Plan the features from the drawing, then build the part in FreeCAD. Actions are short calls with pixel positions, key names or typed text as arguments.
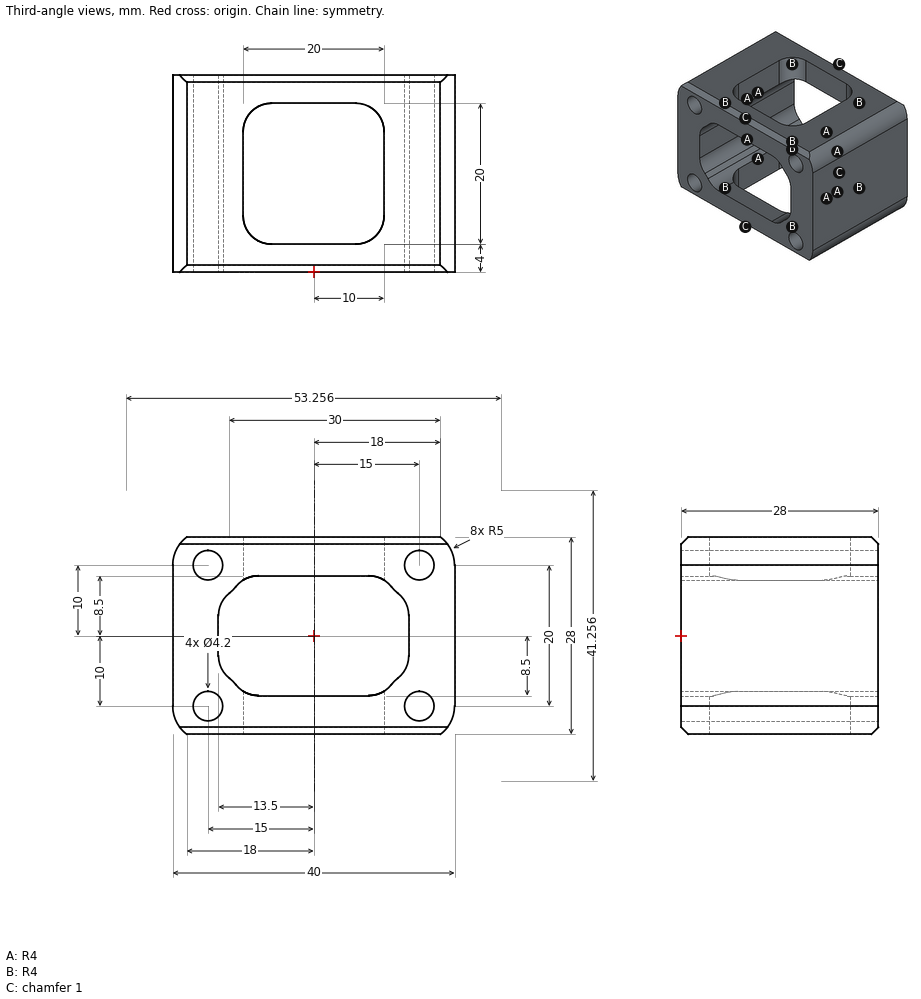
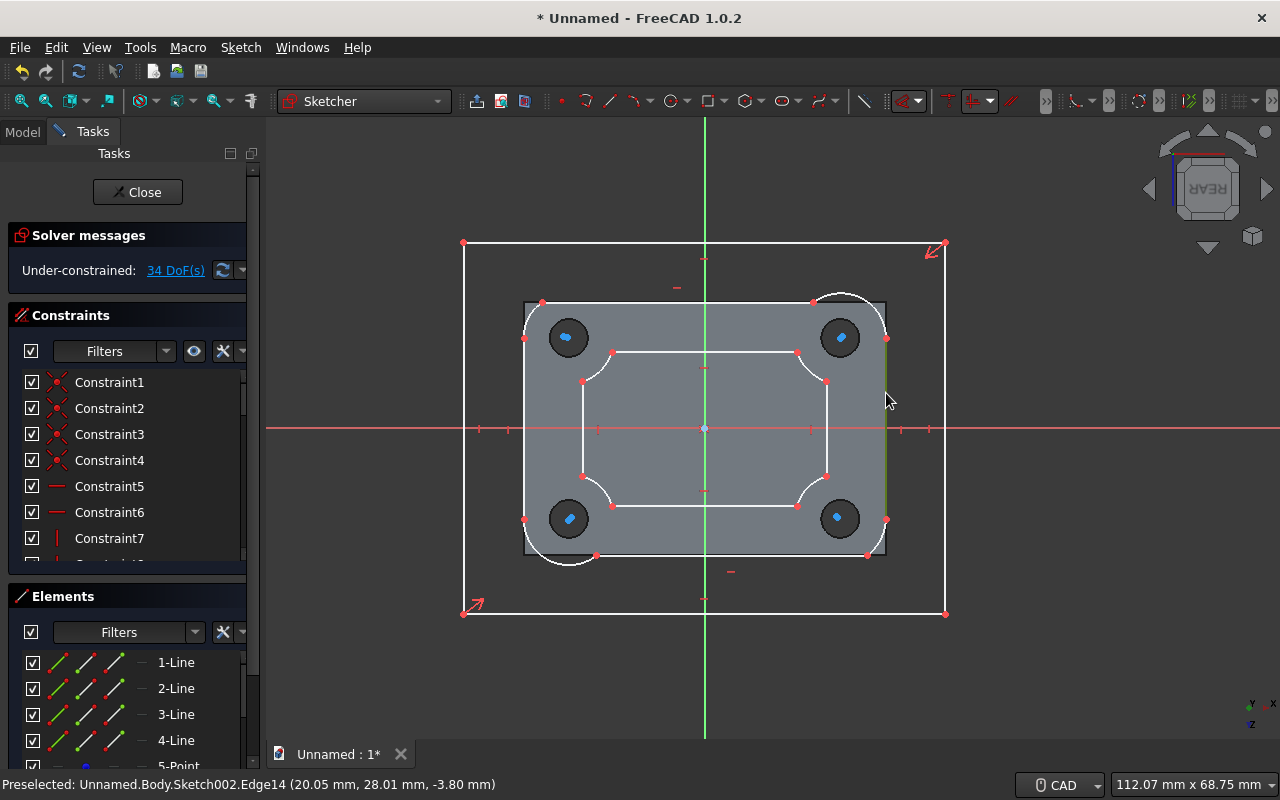
click(876, 547)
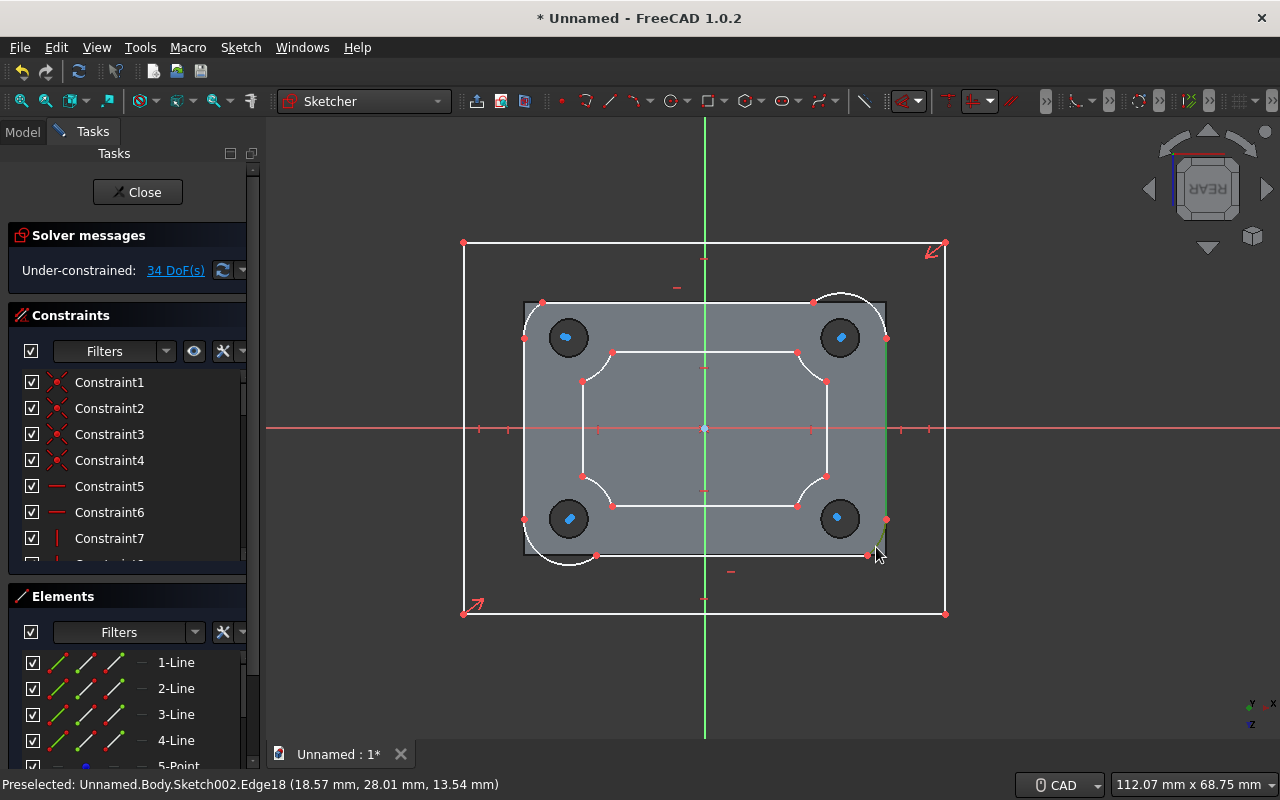
key(t)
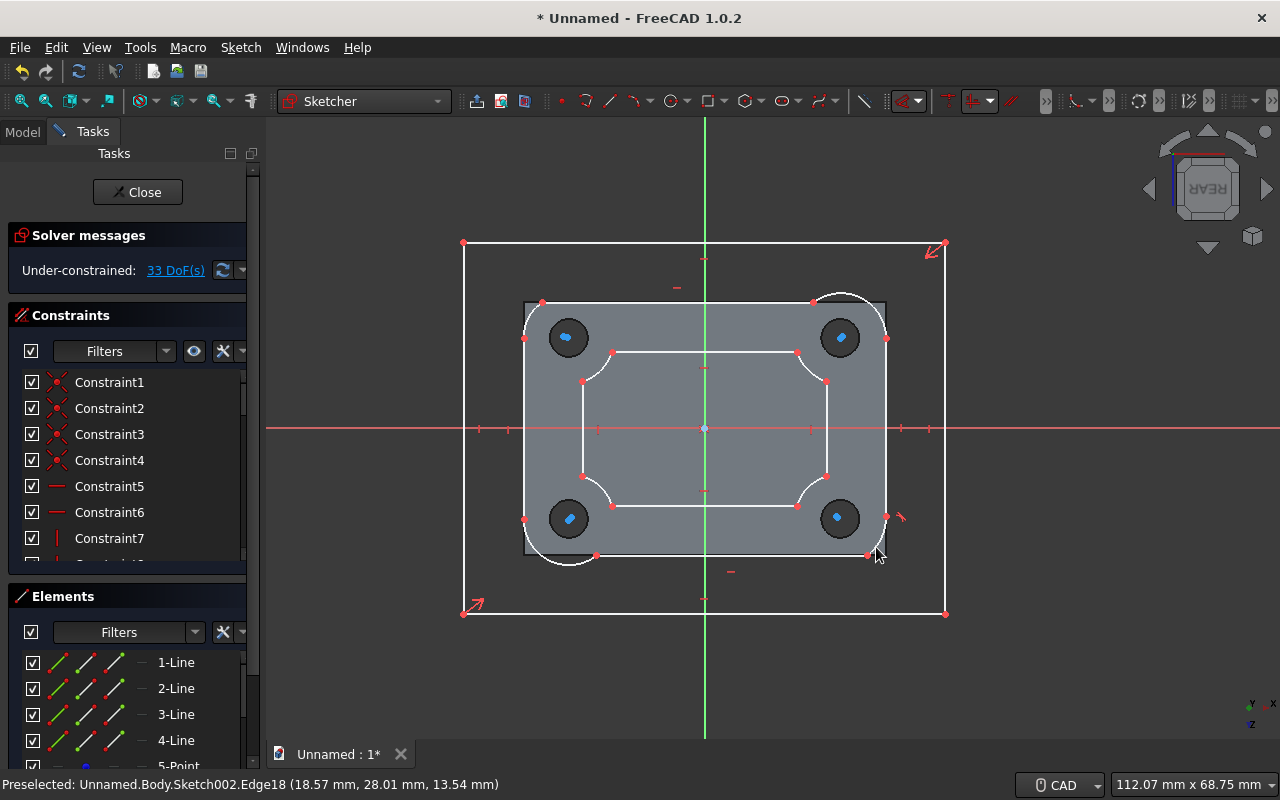
click(886, 392)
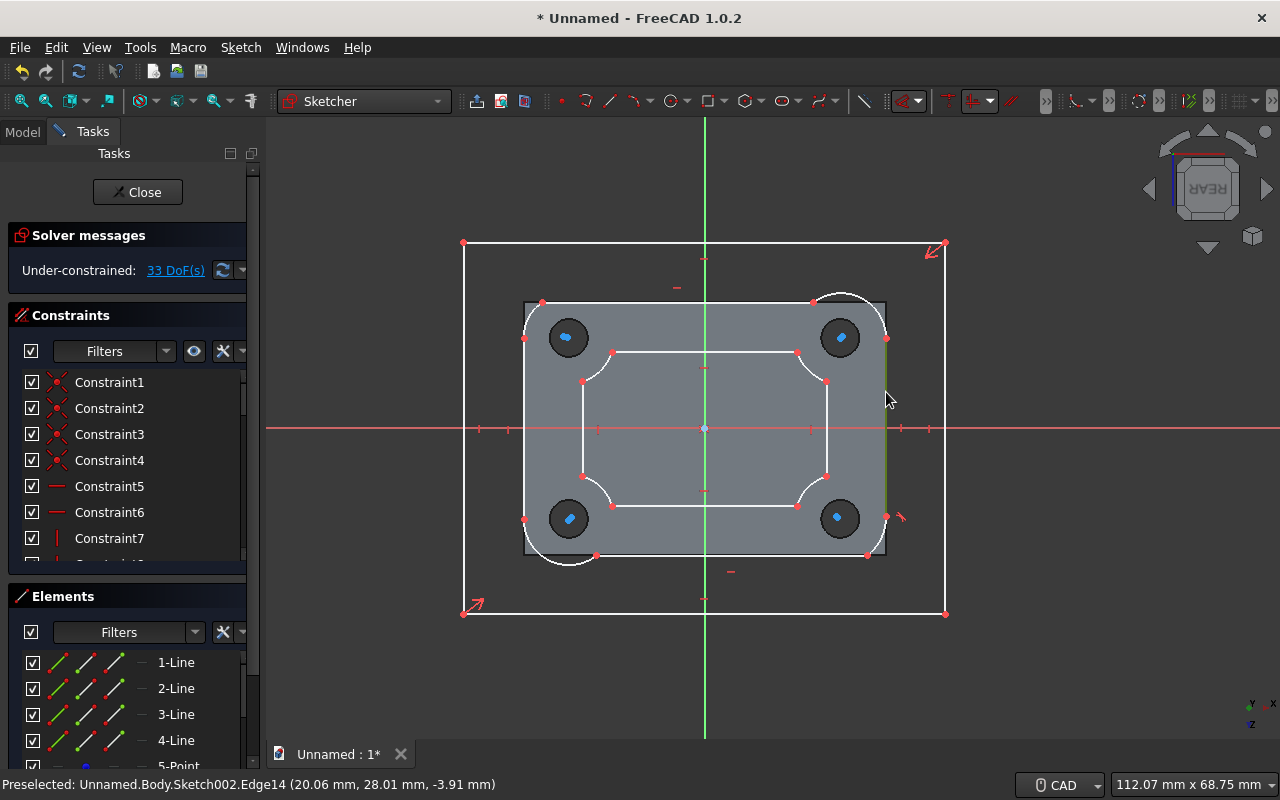
click(877, 311)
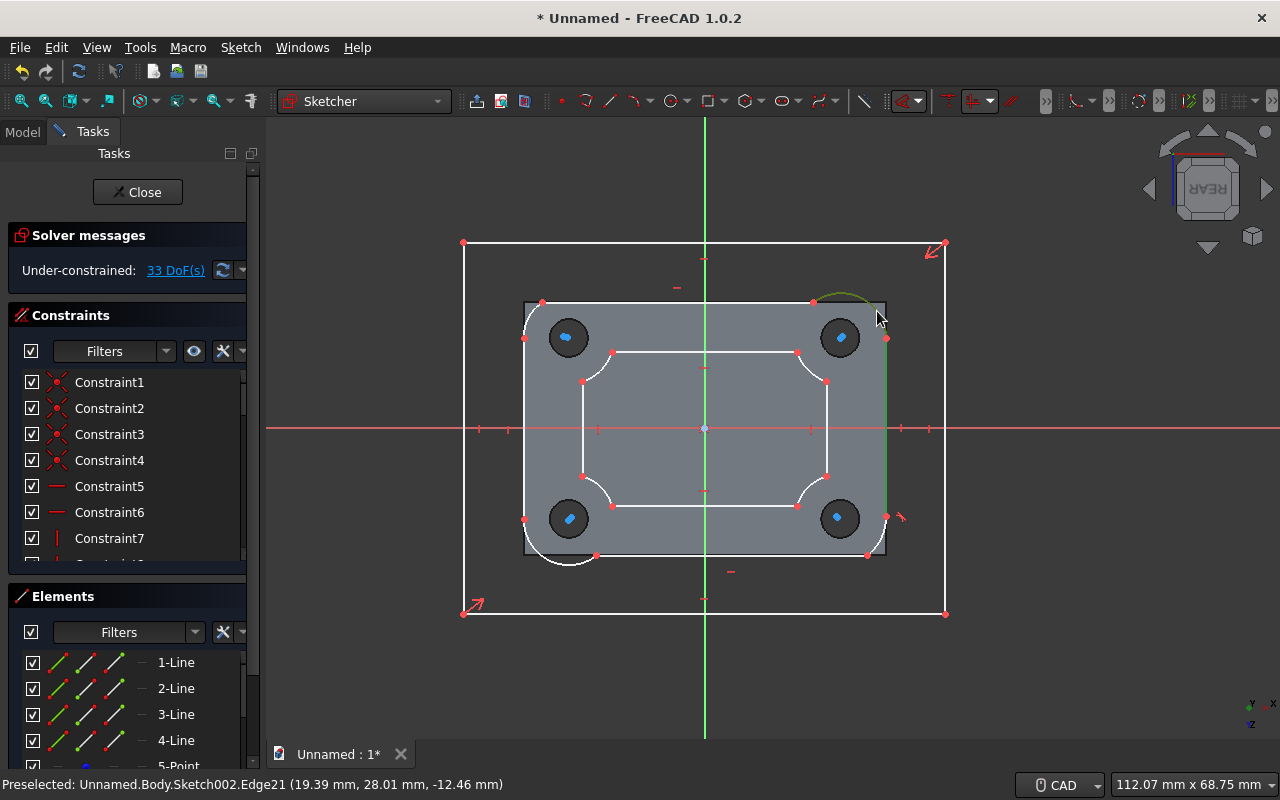
key(t)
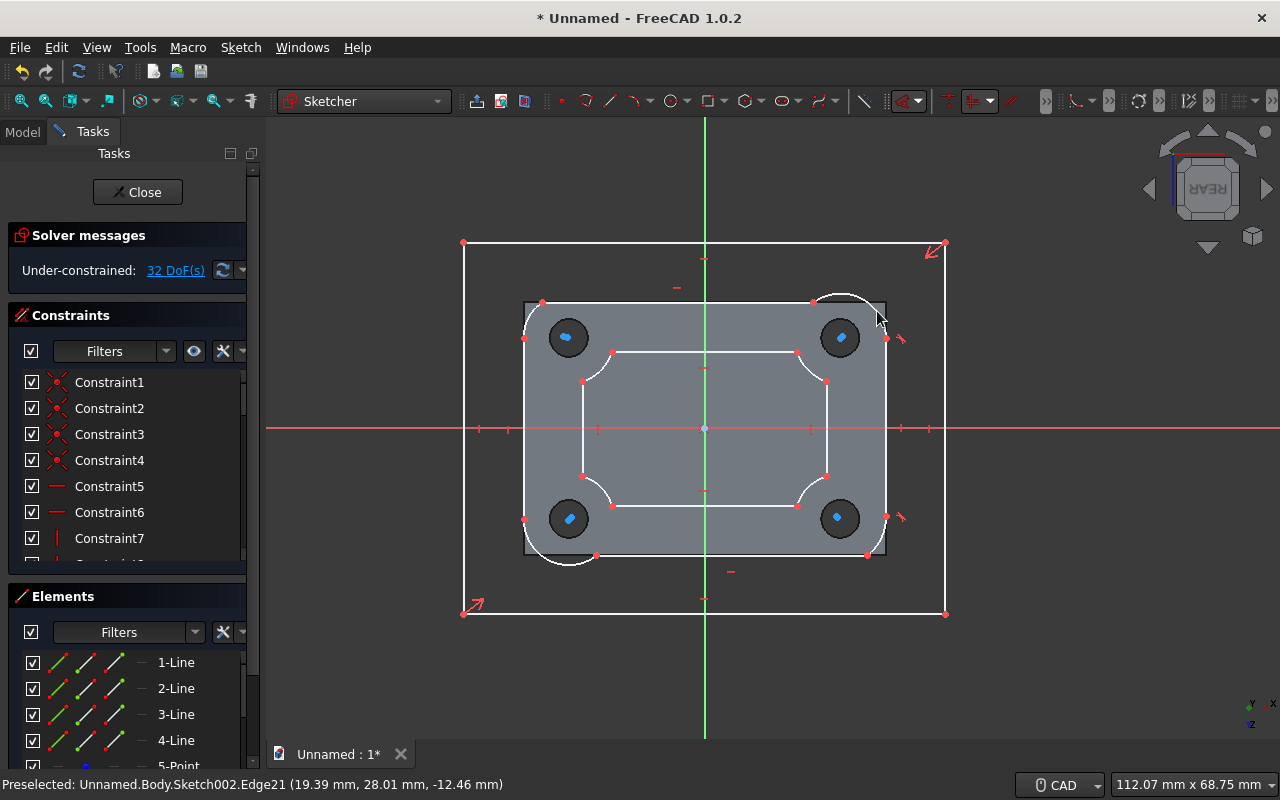
click(524, 466)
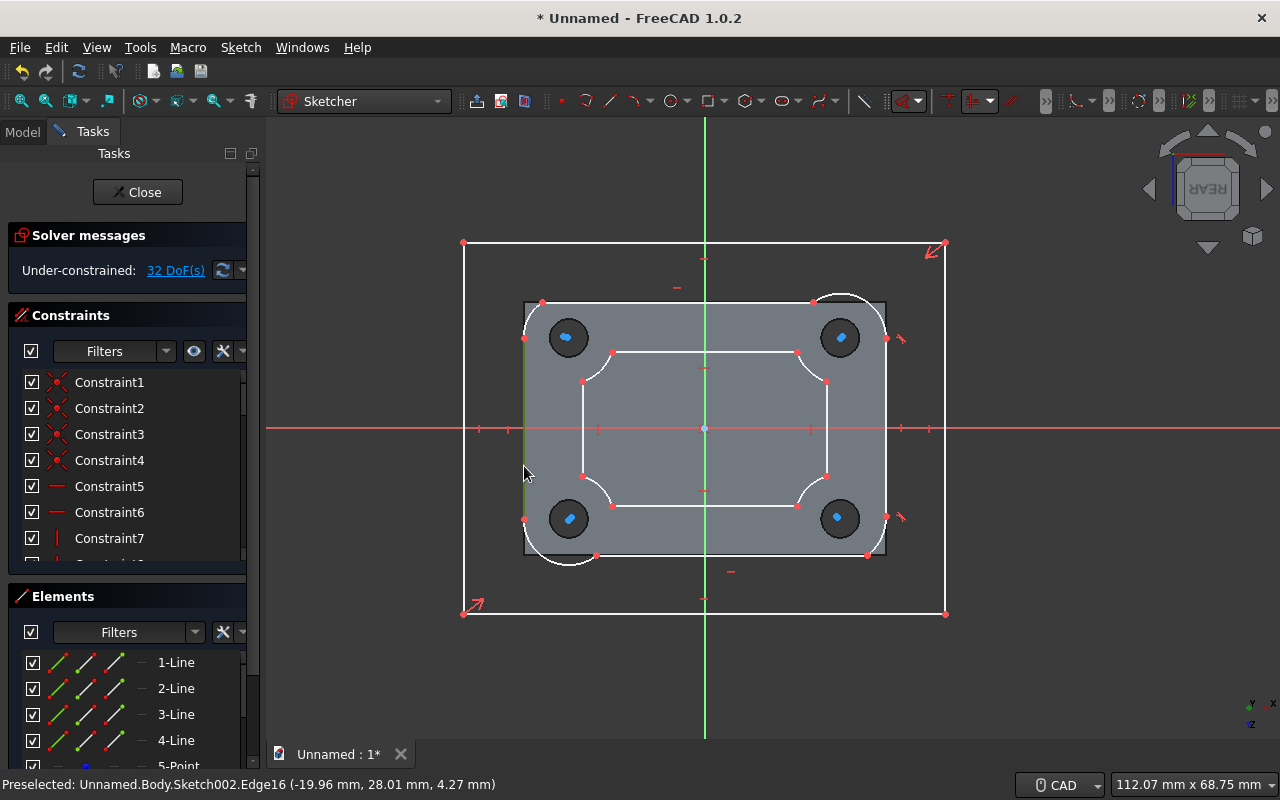
click(534, 548)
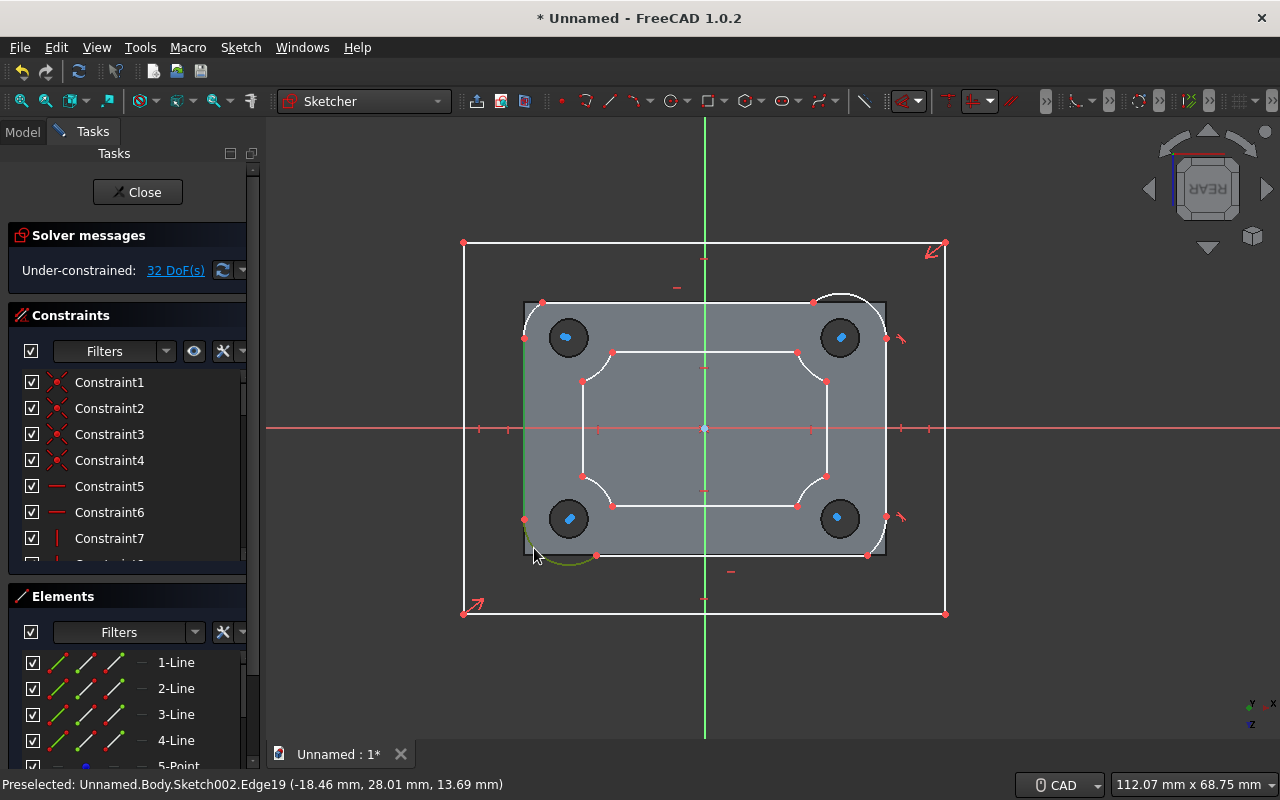
key(t)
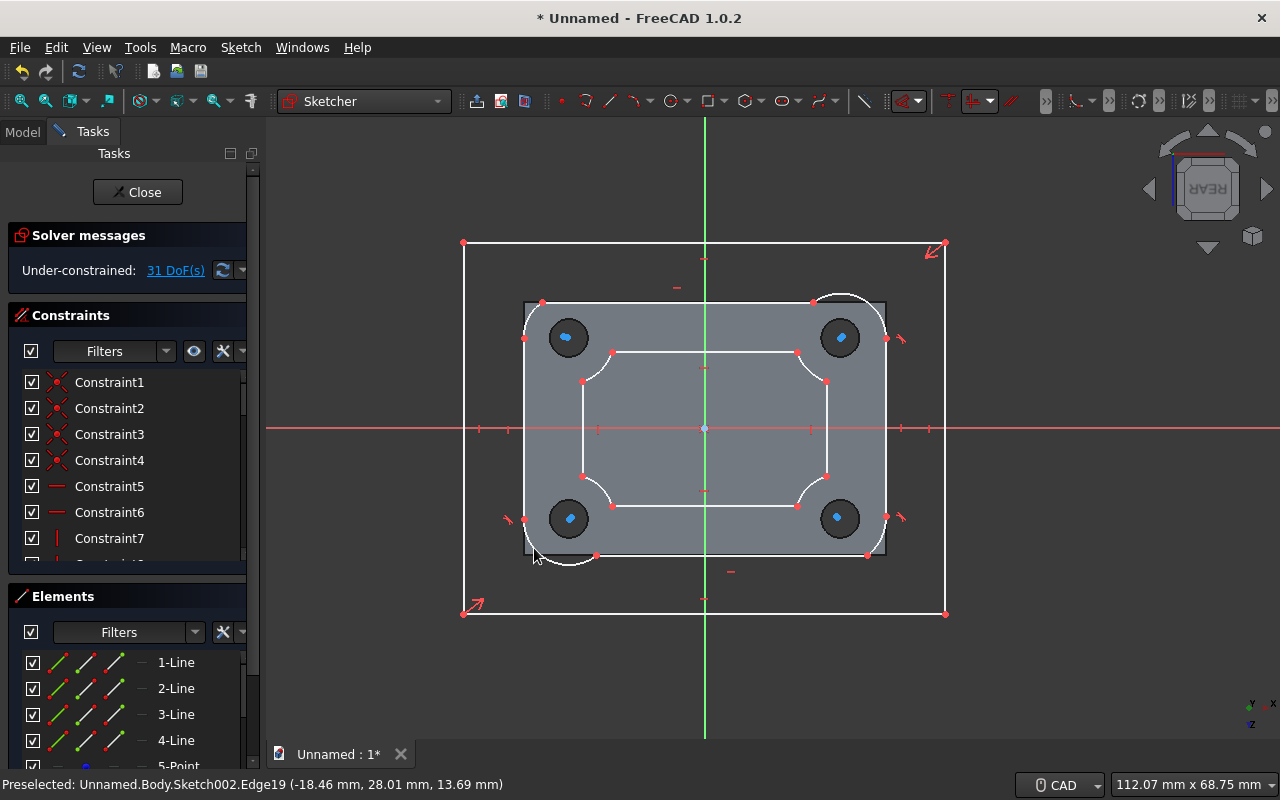
click(524, 466)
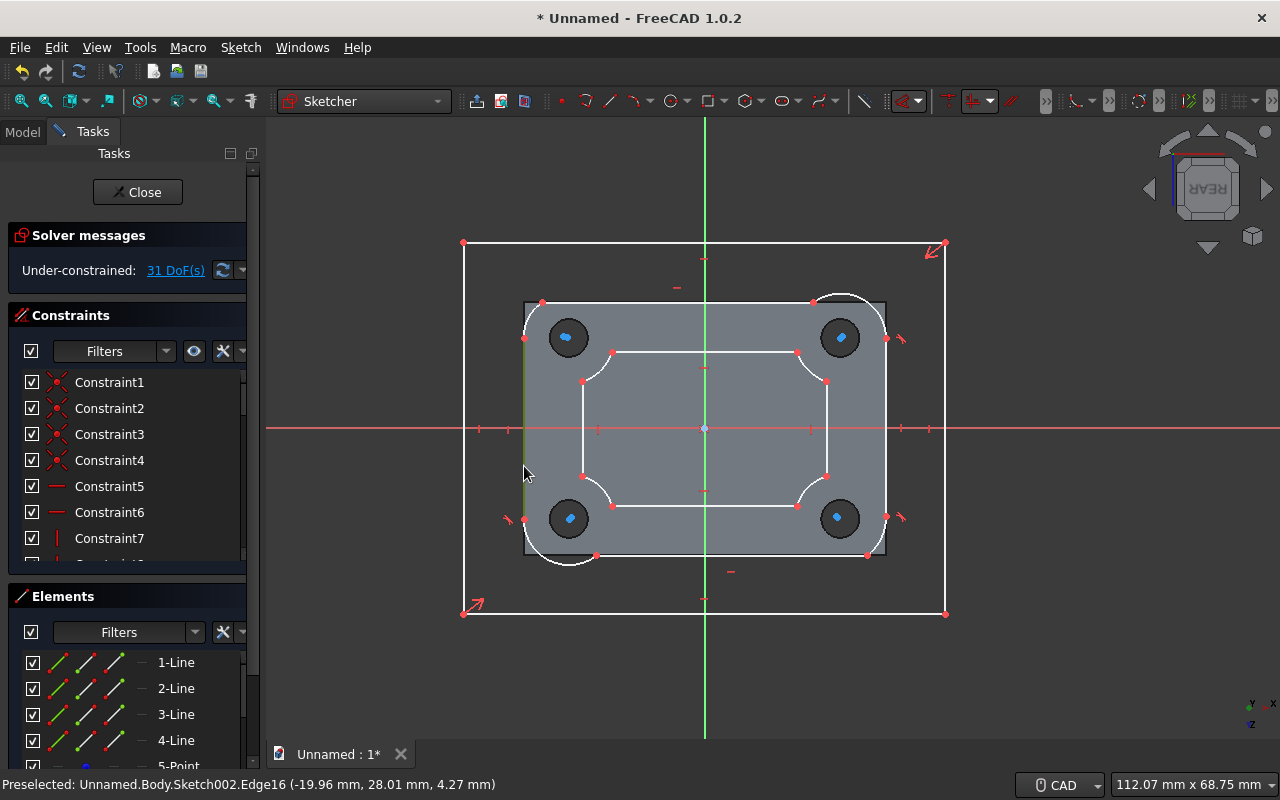
click(533, 311)